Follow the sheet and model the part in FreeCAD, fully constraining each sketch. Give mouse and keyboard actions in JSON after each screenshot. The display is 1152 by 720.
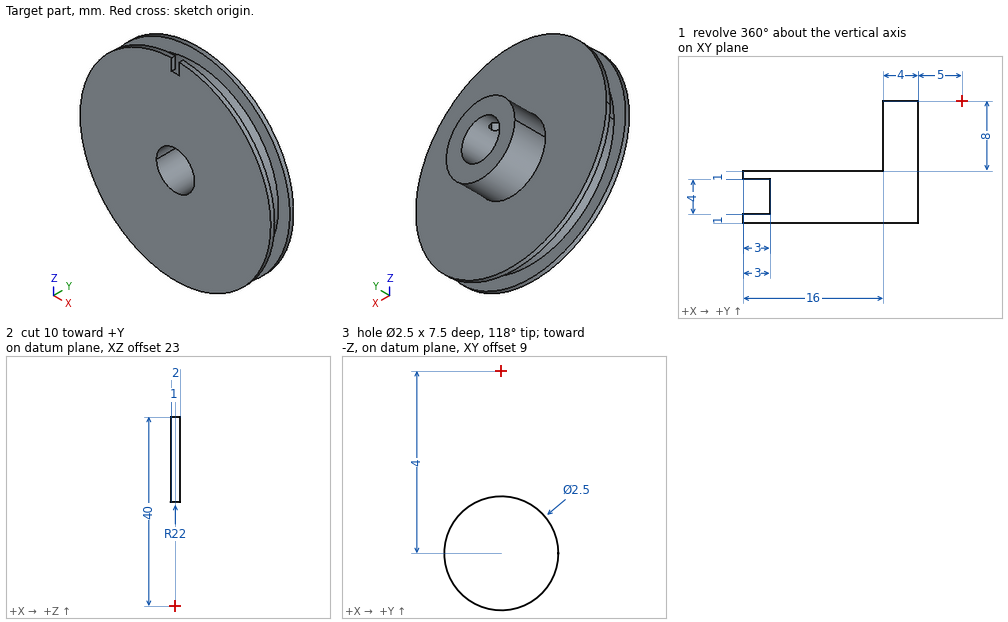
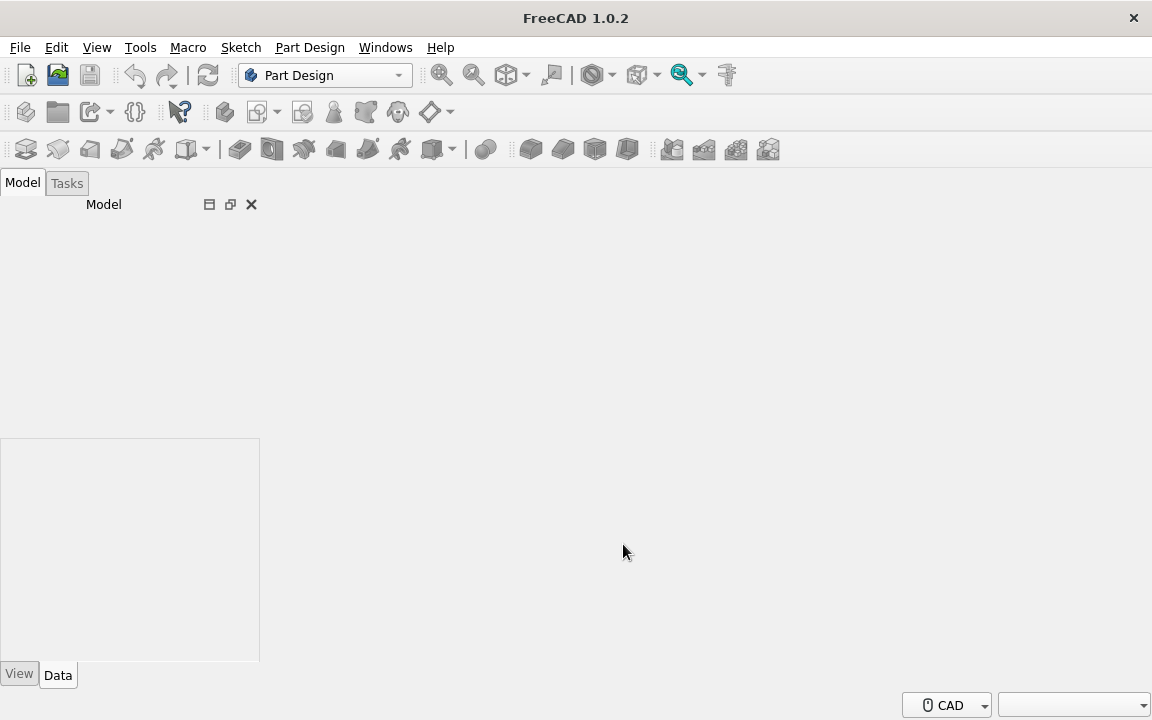
{"action": "left_click", "coordinate": [26, 76]}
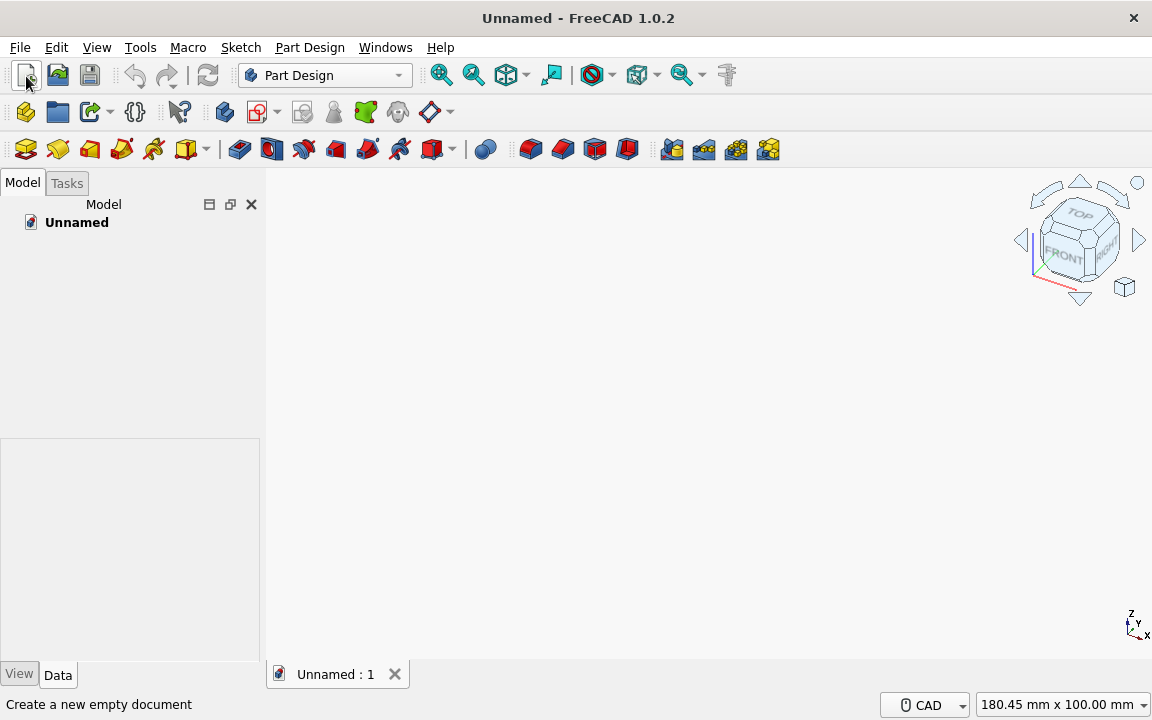
{"action": "left_click", "coordinate": [258, 112]}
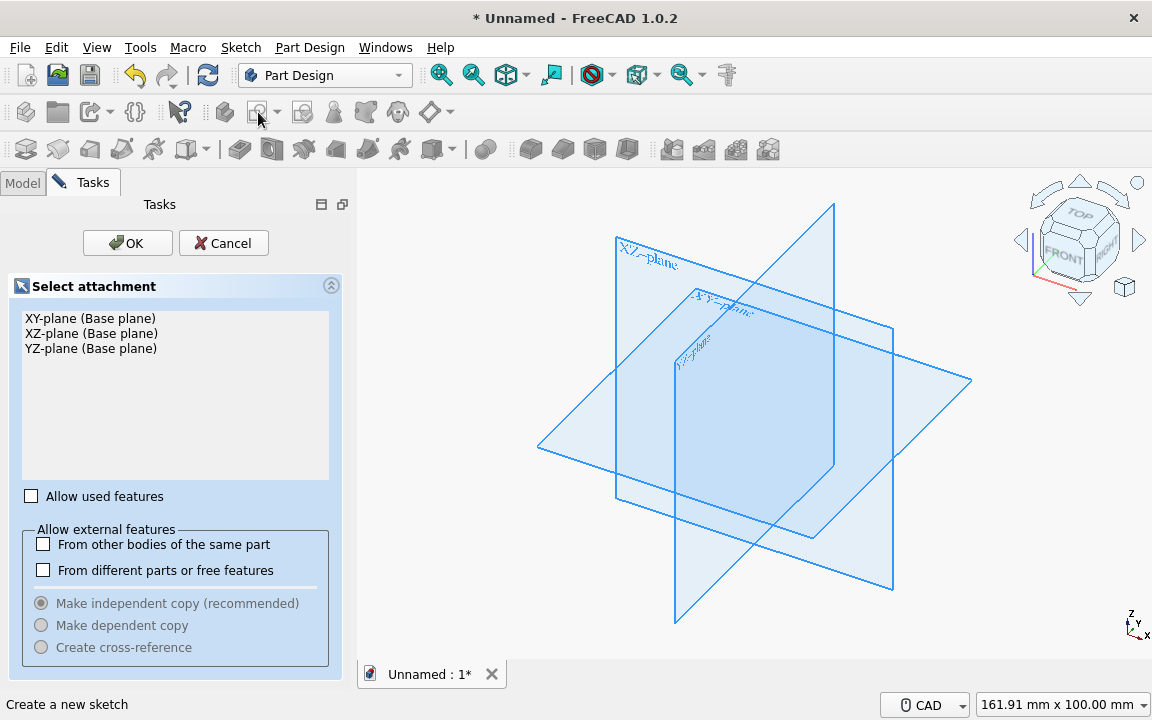
{"action": "left_click", "coordinate": [82, 318]}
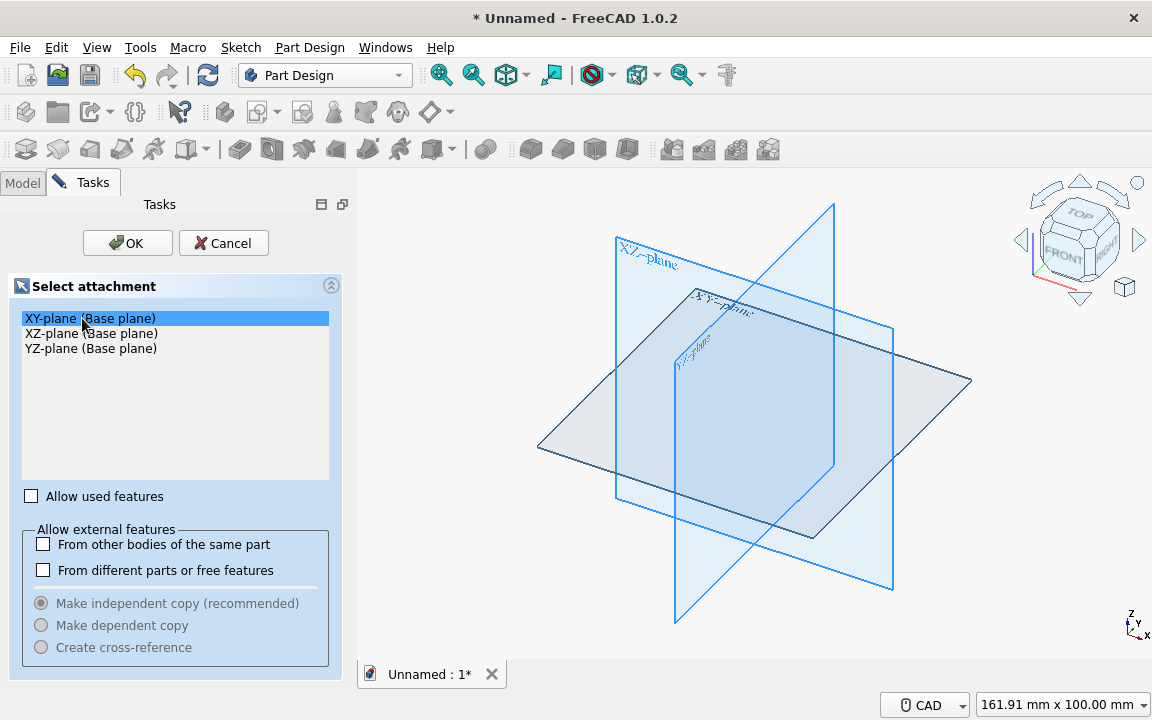
{"action": "left_click", "coordinate": [128, 243]}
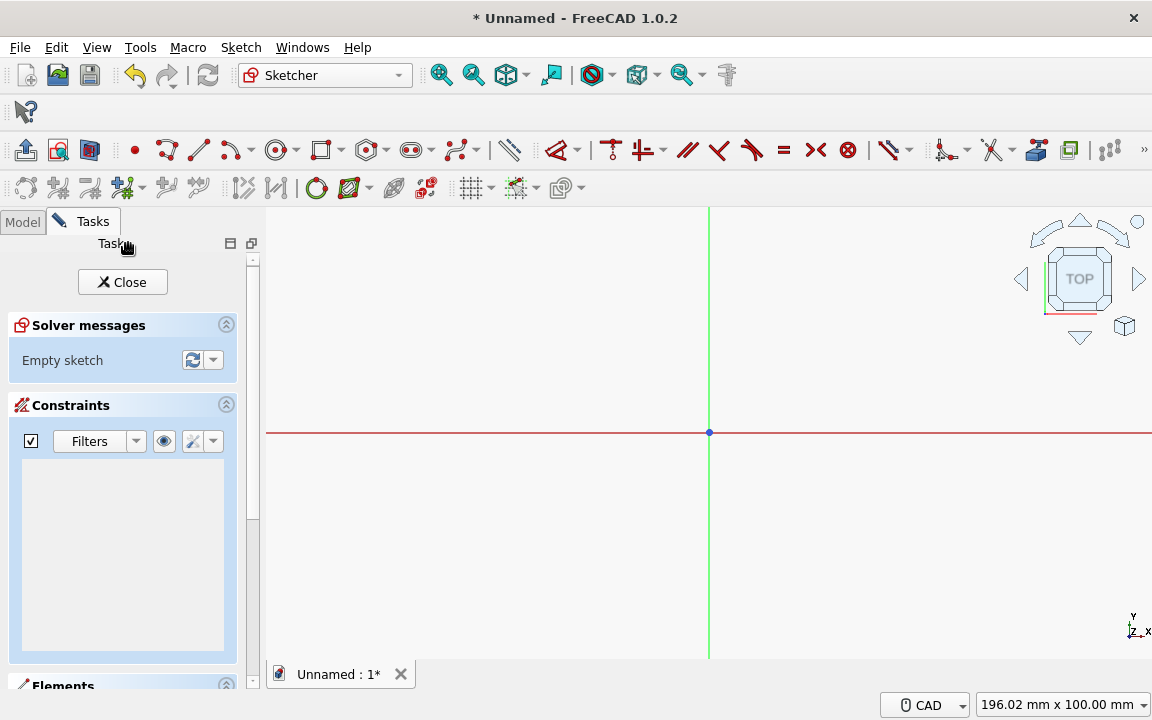
{"action": "scroll", "coordinate": [656, 475], "scroll_direction": "up", "scroll_amount": 7}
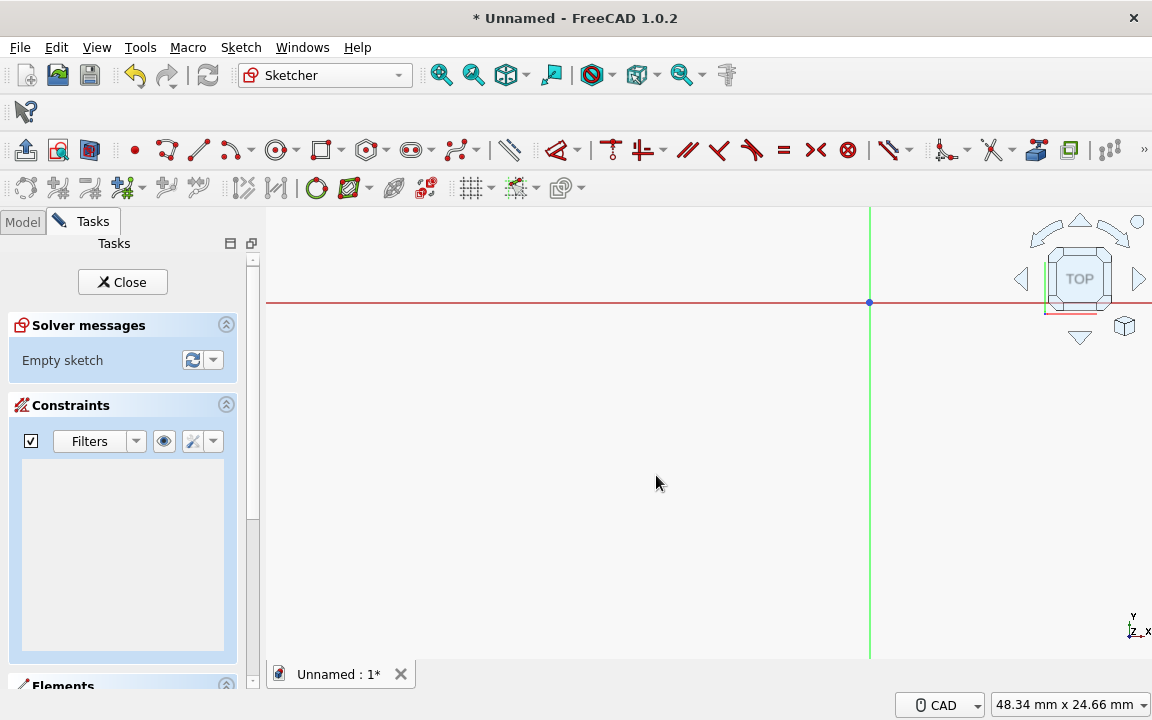
{"action": "key", "text": "g m"}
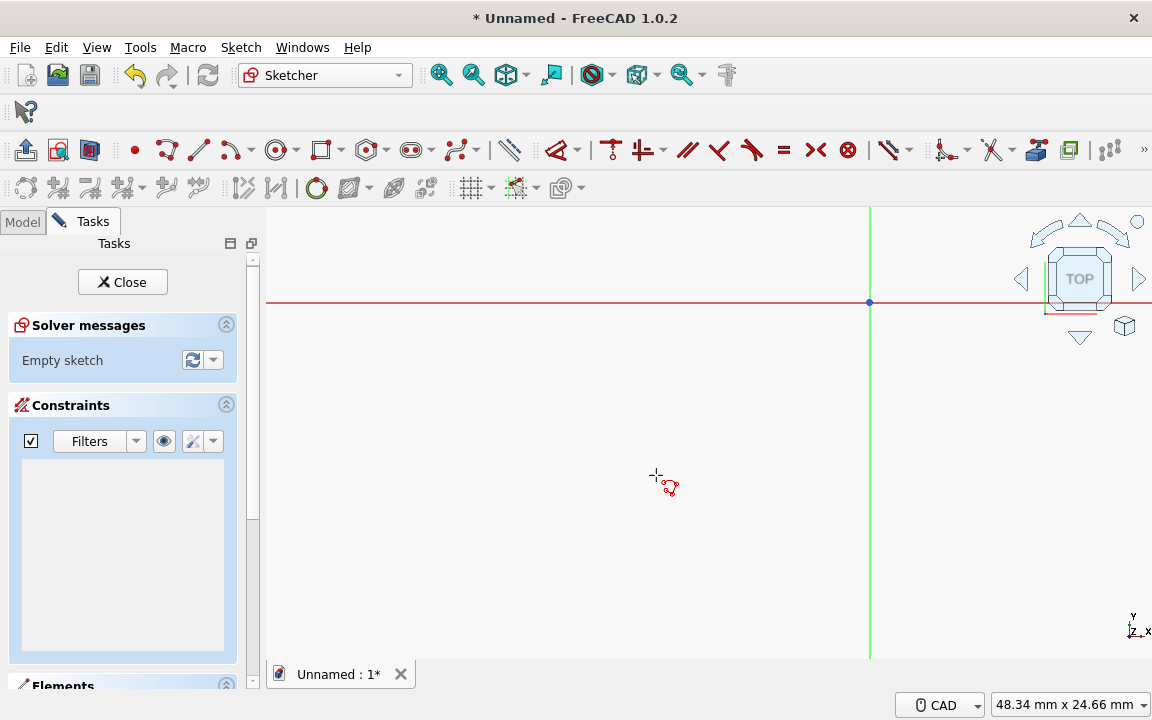
{"action": "left_click", "coordinate": [778, 303]}
{"action": "left_click", "coordinate": [705, 312]}
{"action": "left_click", "coordinate": [705, 450]}
{"action": "left_click", "coordinate": [411, 450]}
{"action": "left_click", "coordinate": [411, 468]}
{"action": "left_click", "coordinate": [466, 468]}
{"action": "left_click", "coordinate": [466, 541]}
{"action": "left_click", "coordinate": [411, 541]}
{"action": "left_click", "coordinate": [411, 559]}
{"action": "left_click", "coordinate": [778, 559]}
{"action": "left_click", "coordinate": [778, 303]}
{"action": "key", "text": "Escape"}
{"action": "key", "text": "Escape"}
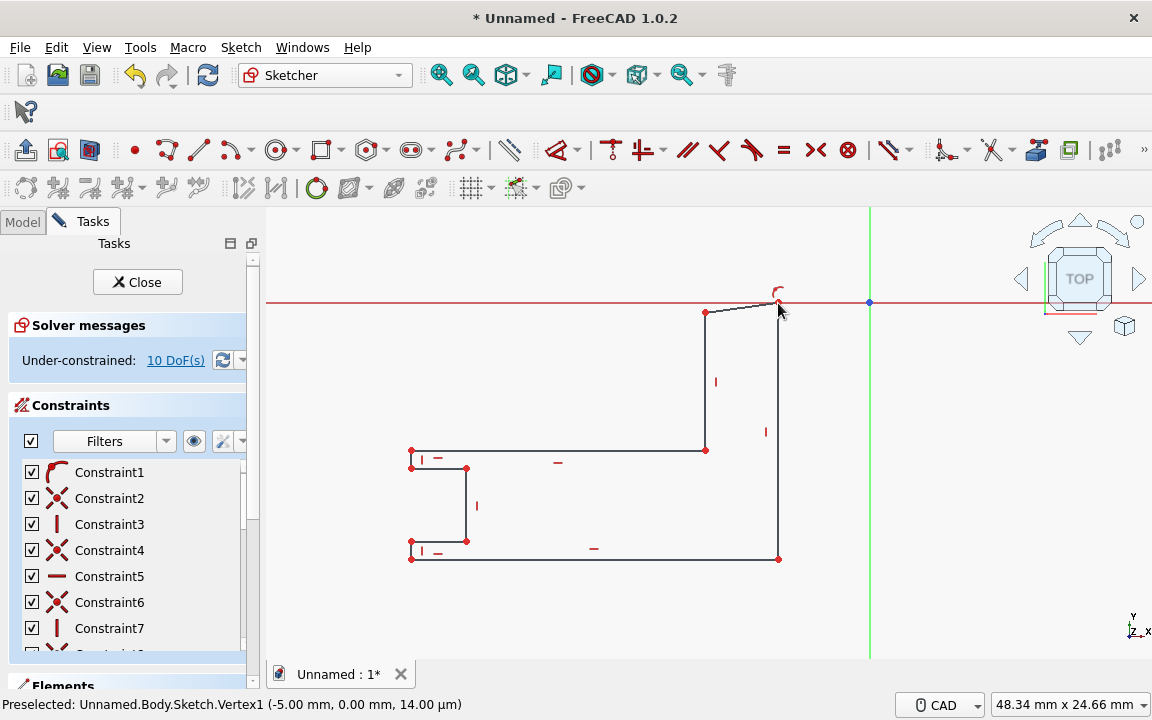
{"action": "left_click", "coordinate": [756, 306]}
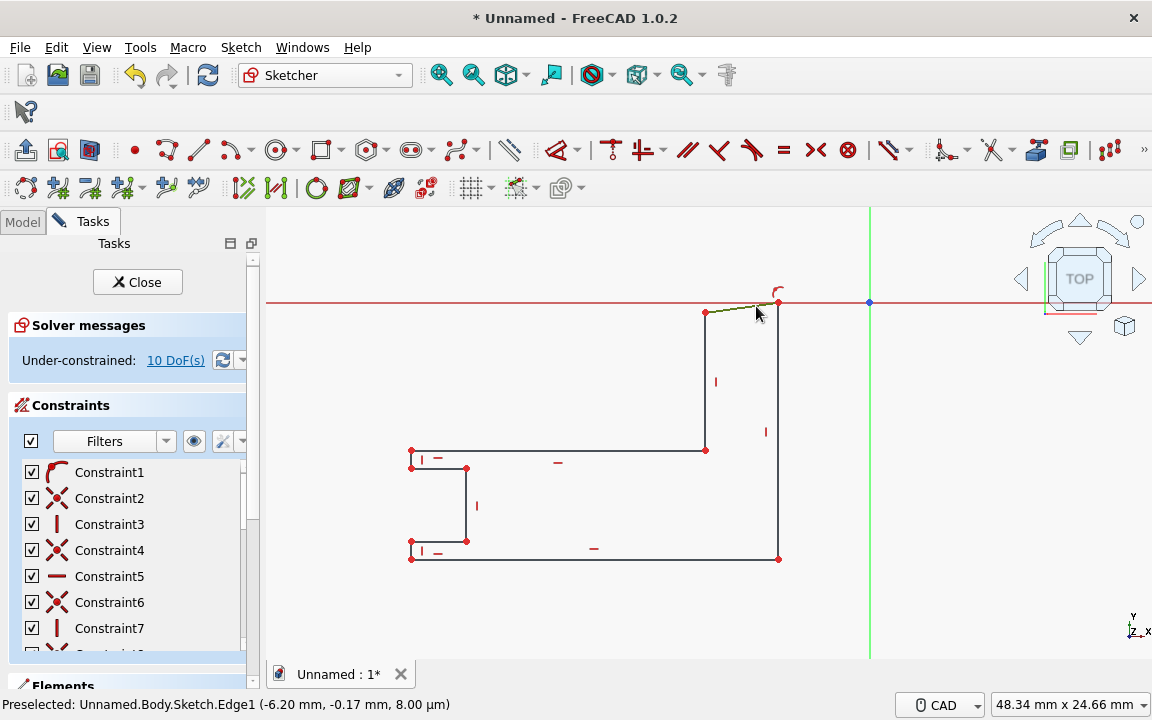
{"action": "key", "text": "h"}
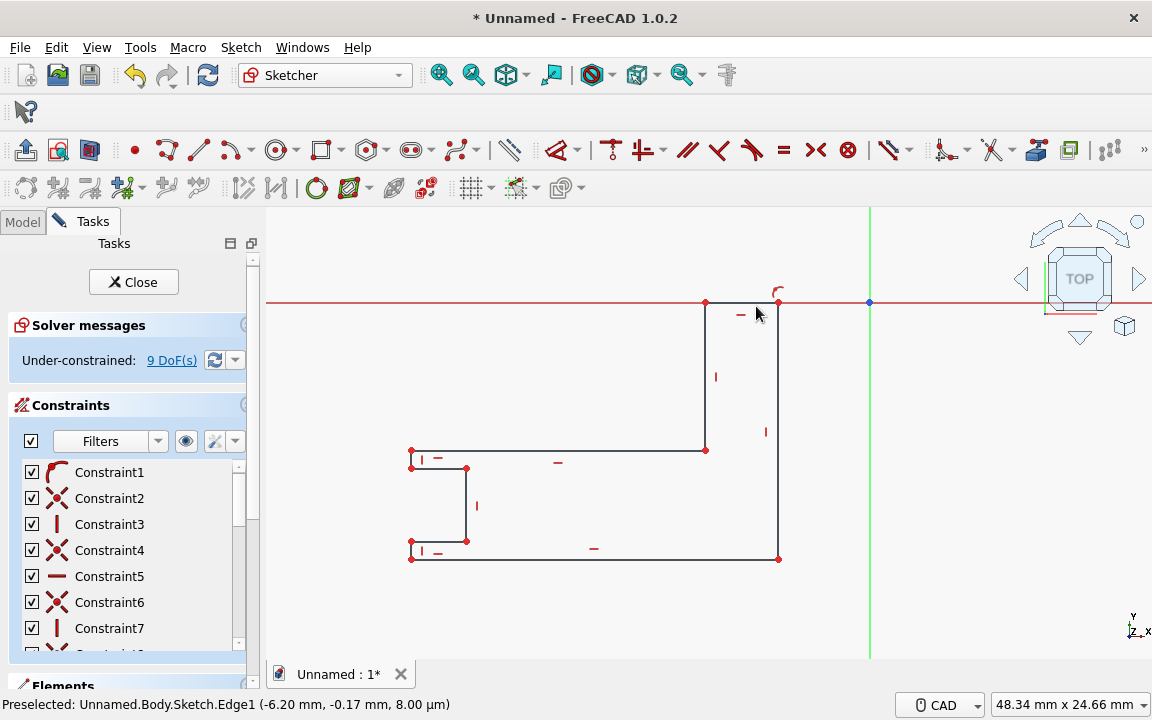
{"action": "left_click", "coordinate": [756, 303]}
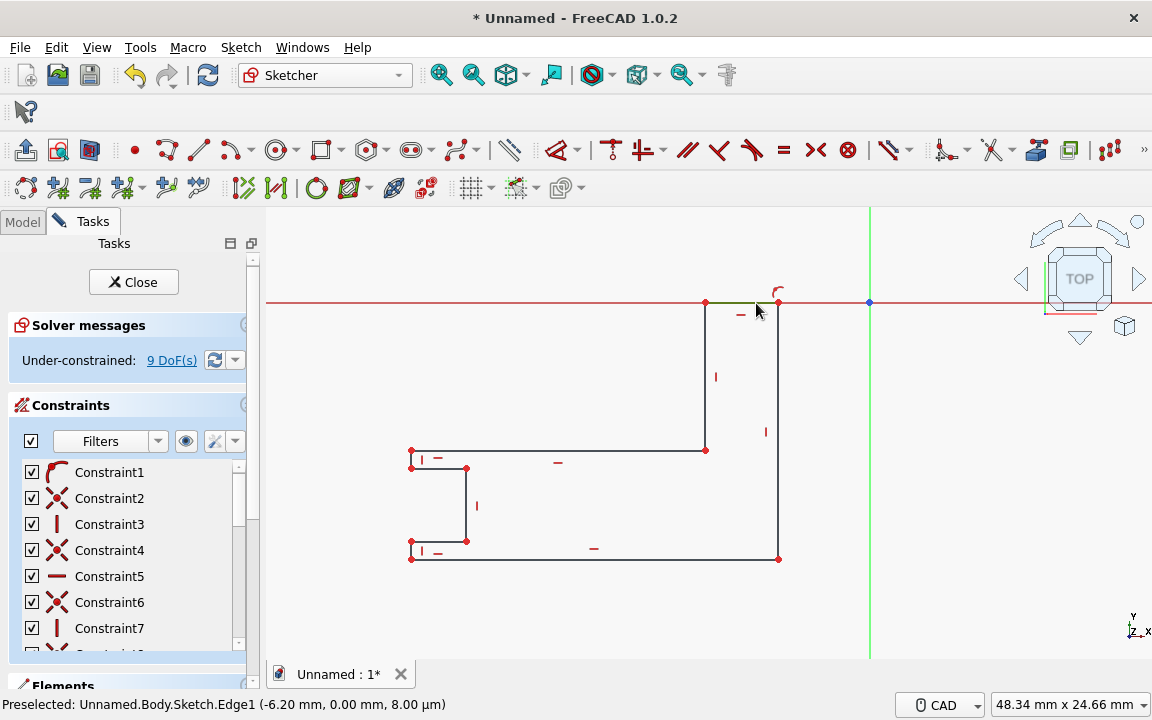
{"action": "left_click", "coordinate": [580, 150]}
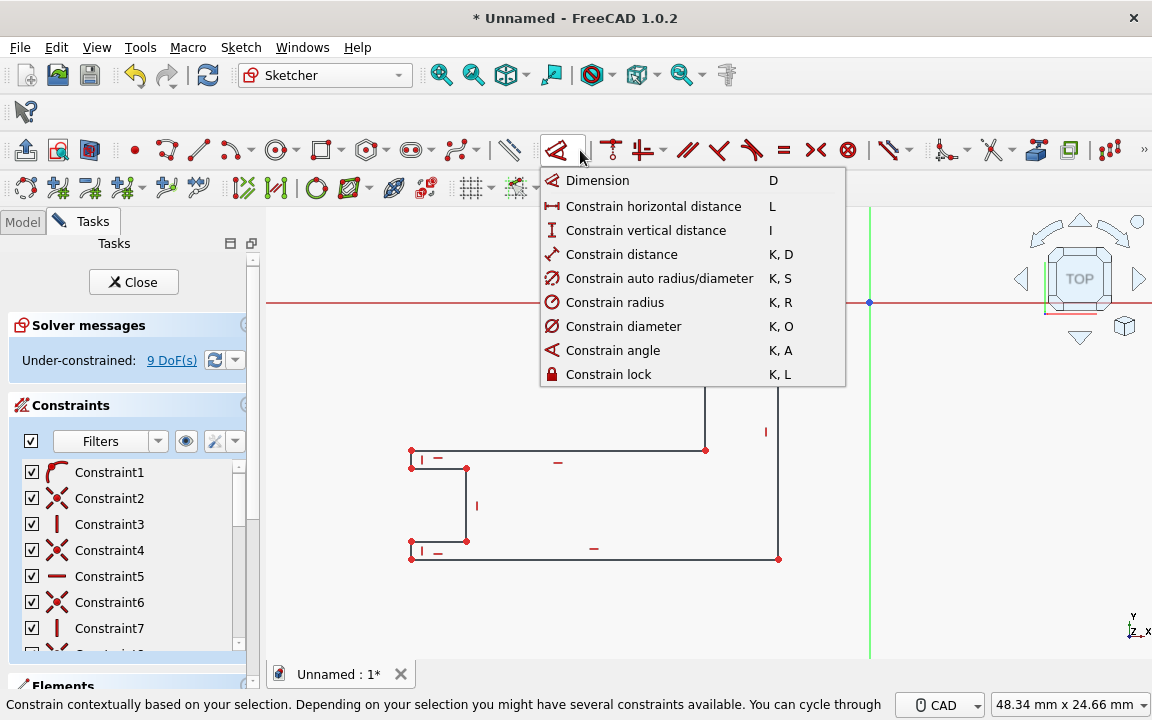
{"action": "left_click", "coordinate": [693, 206]}